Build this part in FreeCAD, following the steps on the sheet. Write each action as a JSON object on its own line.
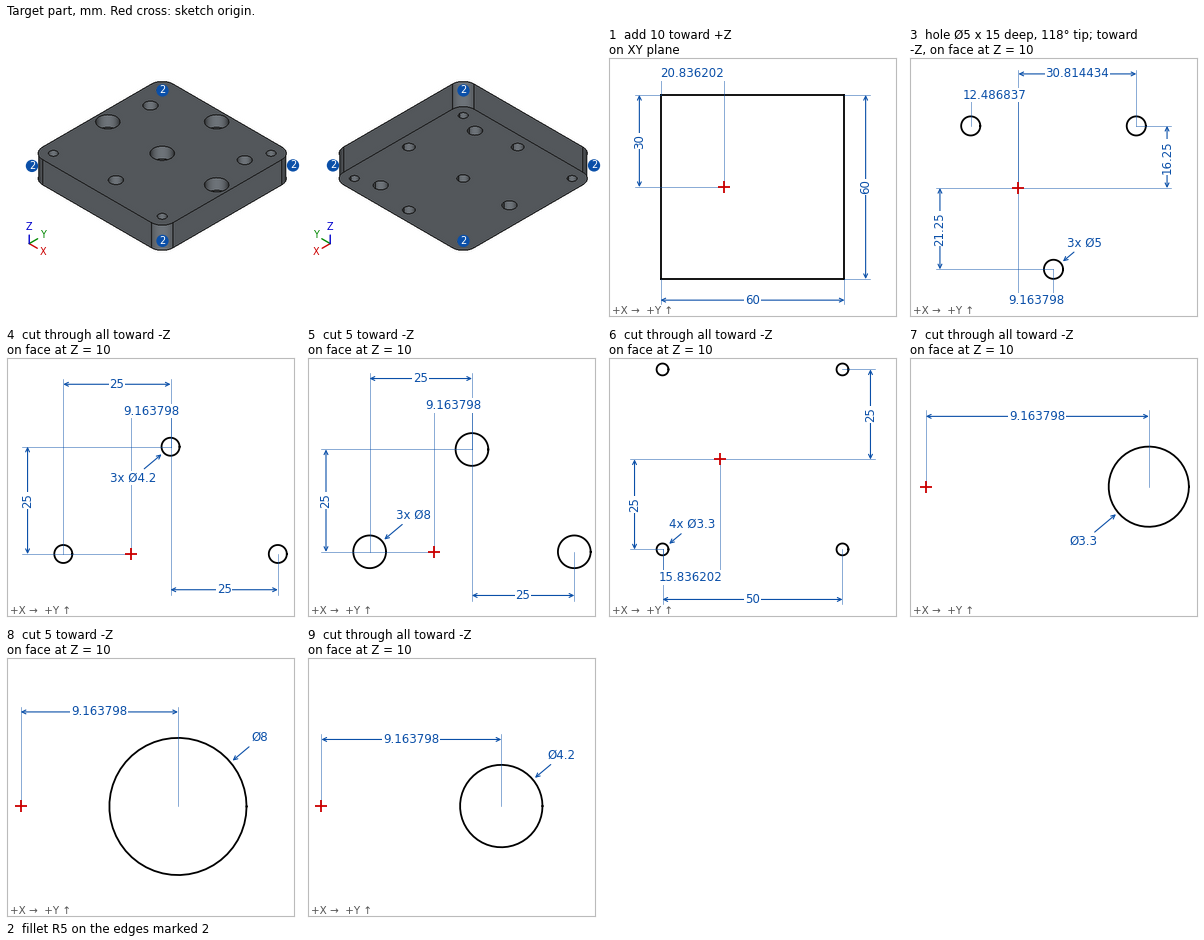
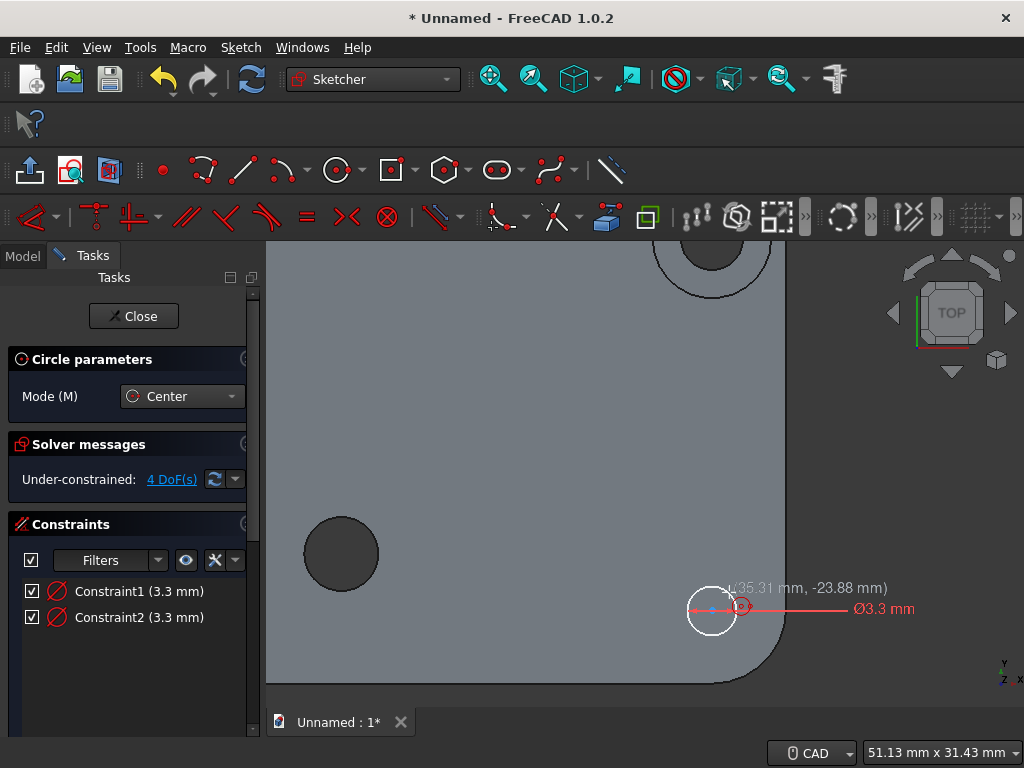
{"action": "scroll", "coordinate": [713, 611], "scroll_direction": "down", "scroll_amount": 5}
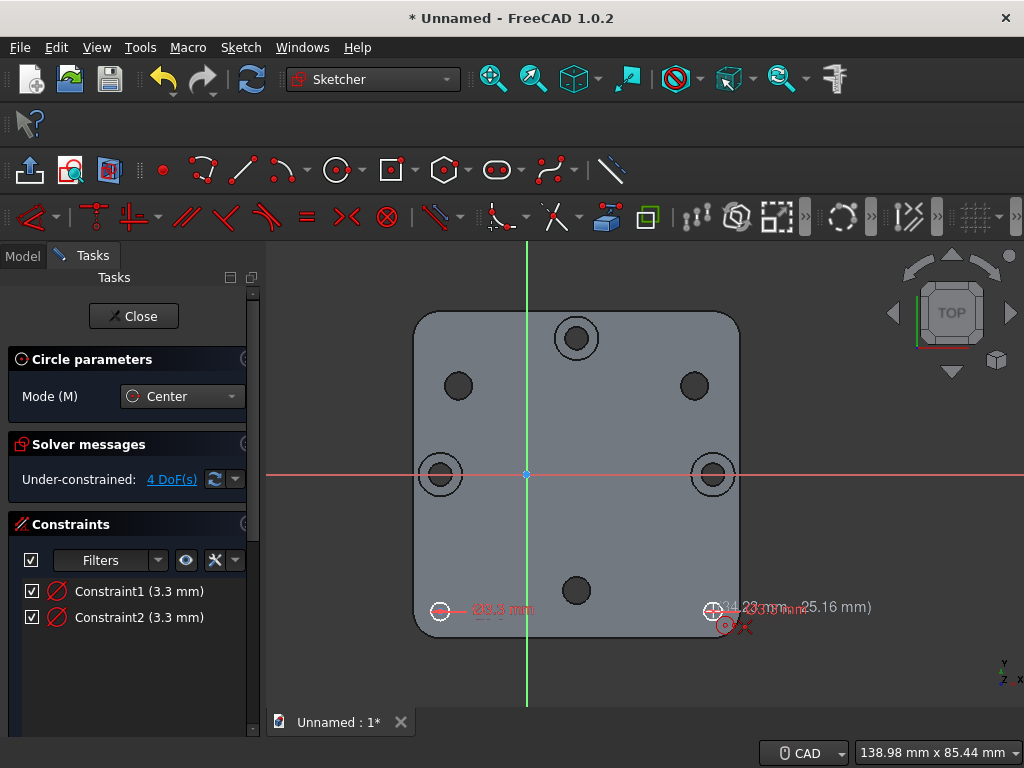
{"action": "scroll", "coordinate": [713, 338], "scroll_direction": "up", "scroll_amount": 5}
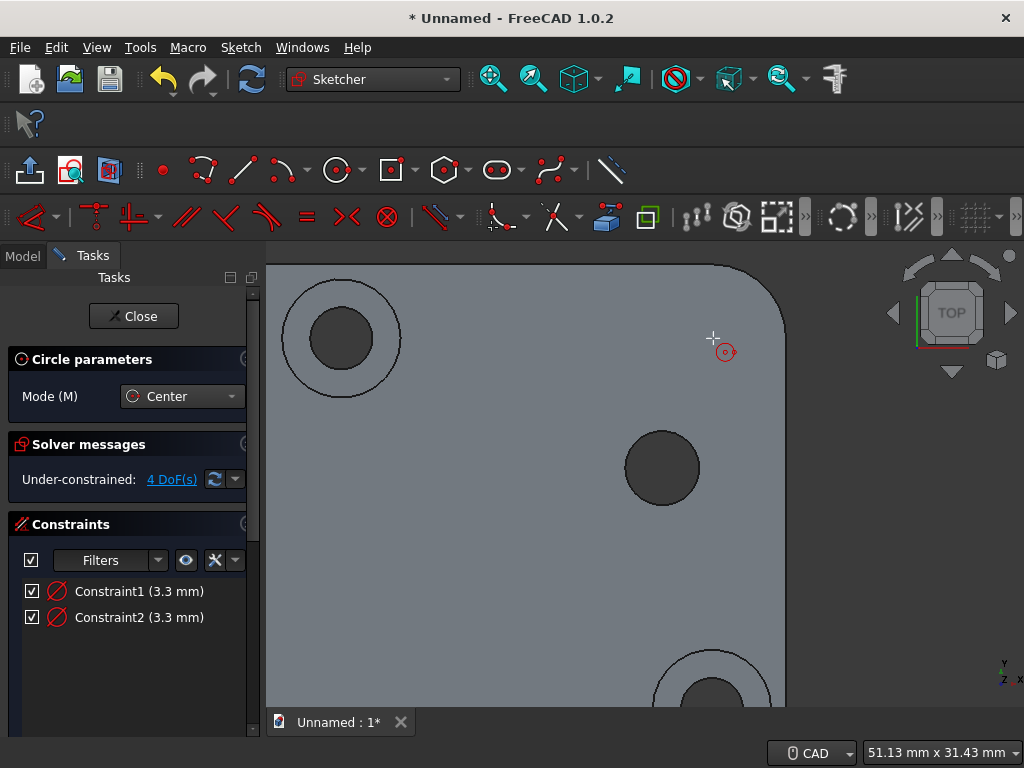
{"action": "left_click", "coordinate": [712, 338]}
{"action": "mouse_move", "coordinate": [729, 321]}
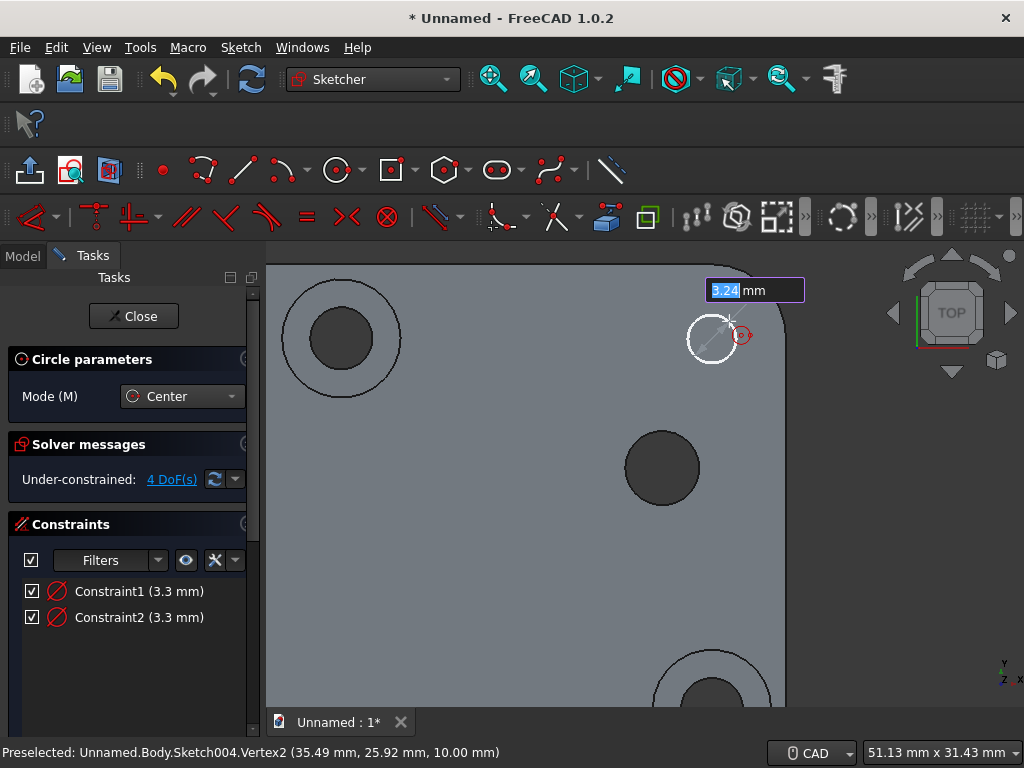
{"action": "type", "text": "3.3"}
{"action": "key", "text": "Return"}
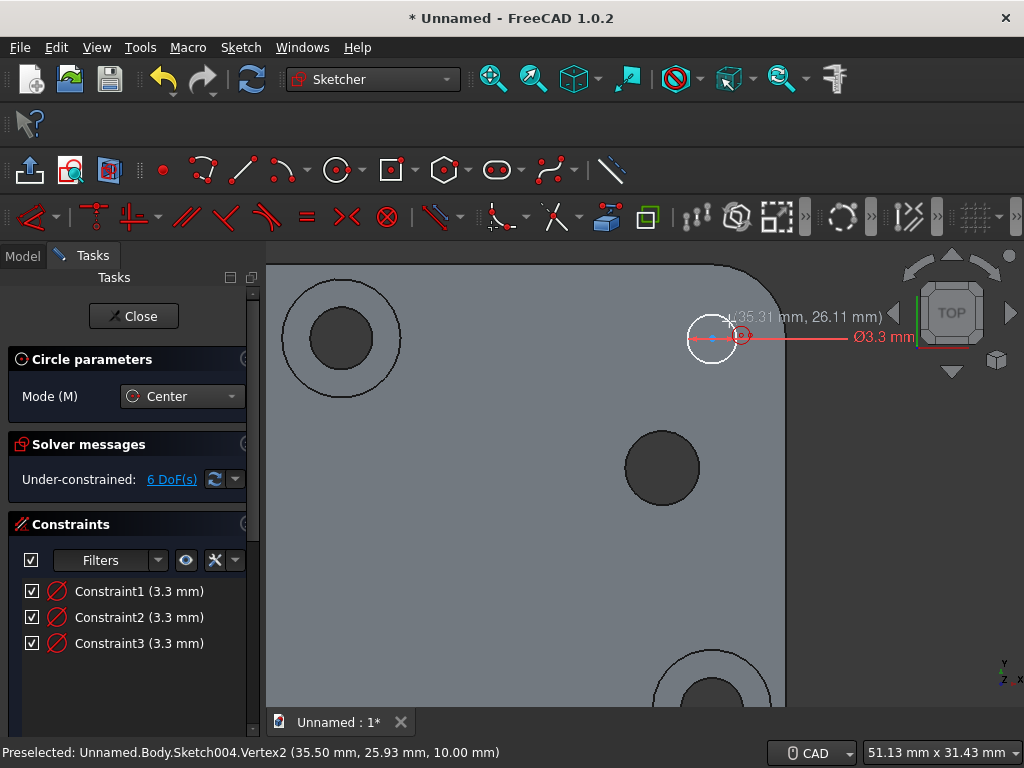
{"action": "scroll", "coordinate": [713, 337], "scroll_direction": "down", "scroll_amount": 5}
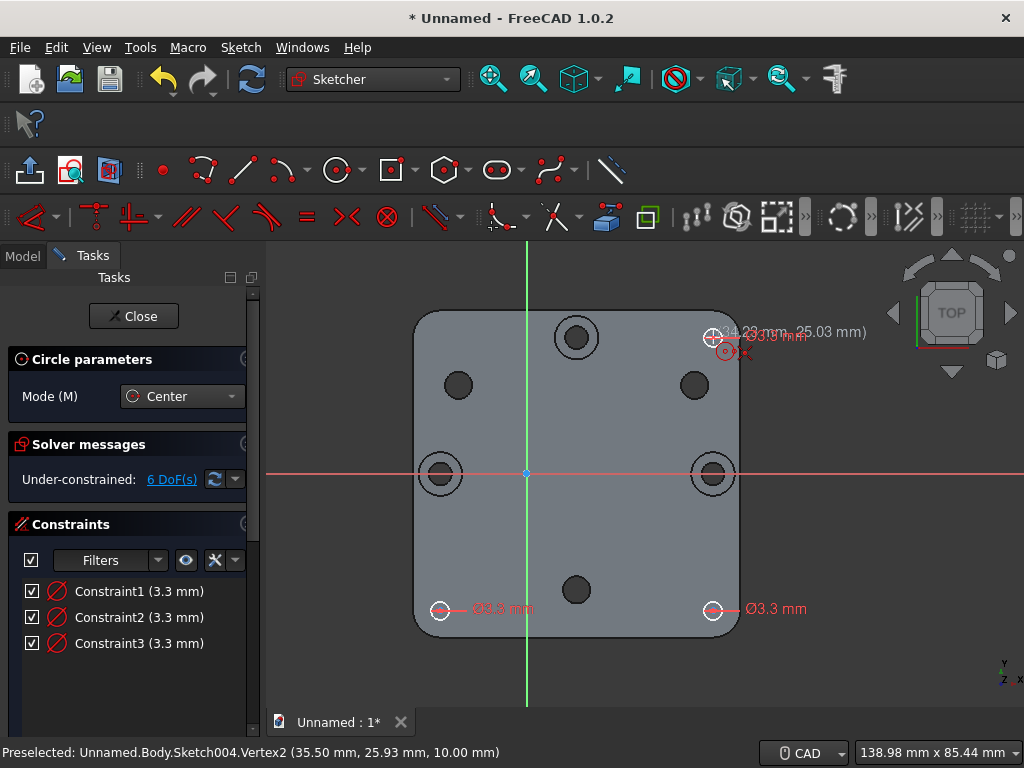
{"action": "scroll", "coordinate": [440, 338], "scroll_direction": "up", "scroll_amount": 5}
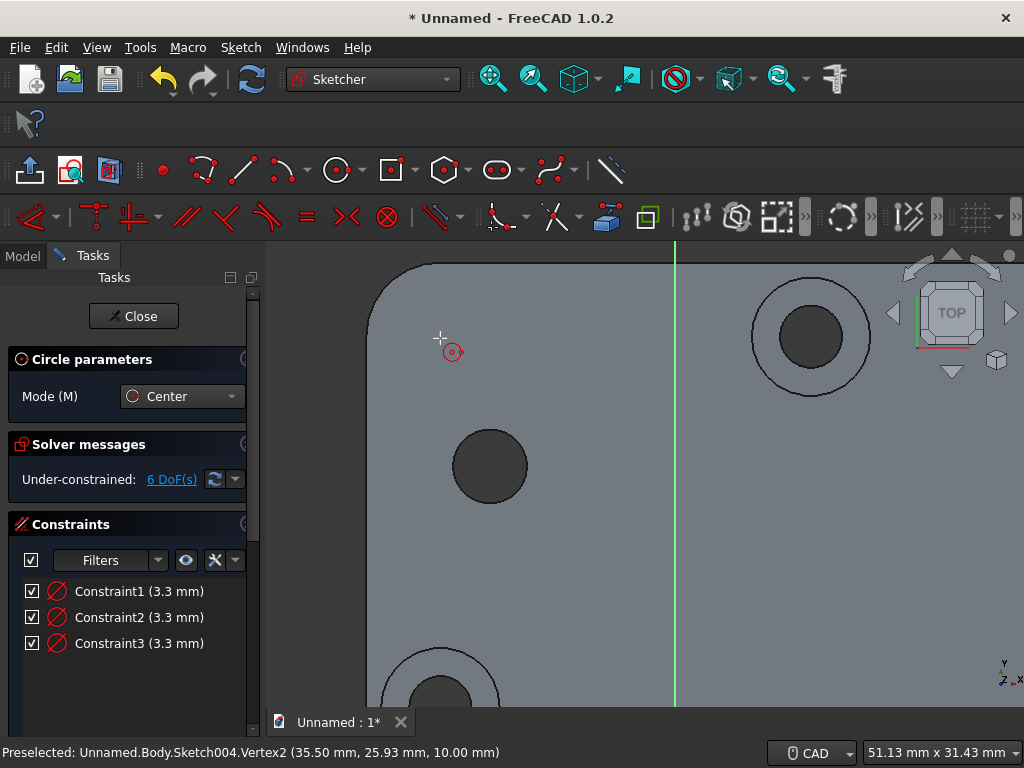
{"action": "left_click", "coordinate": [440, 337]}
{"action": "mouse_move", "coordinate": [458, 319]}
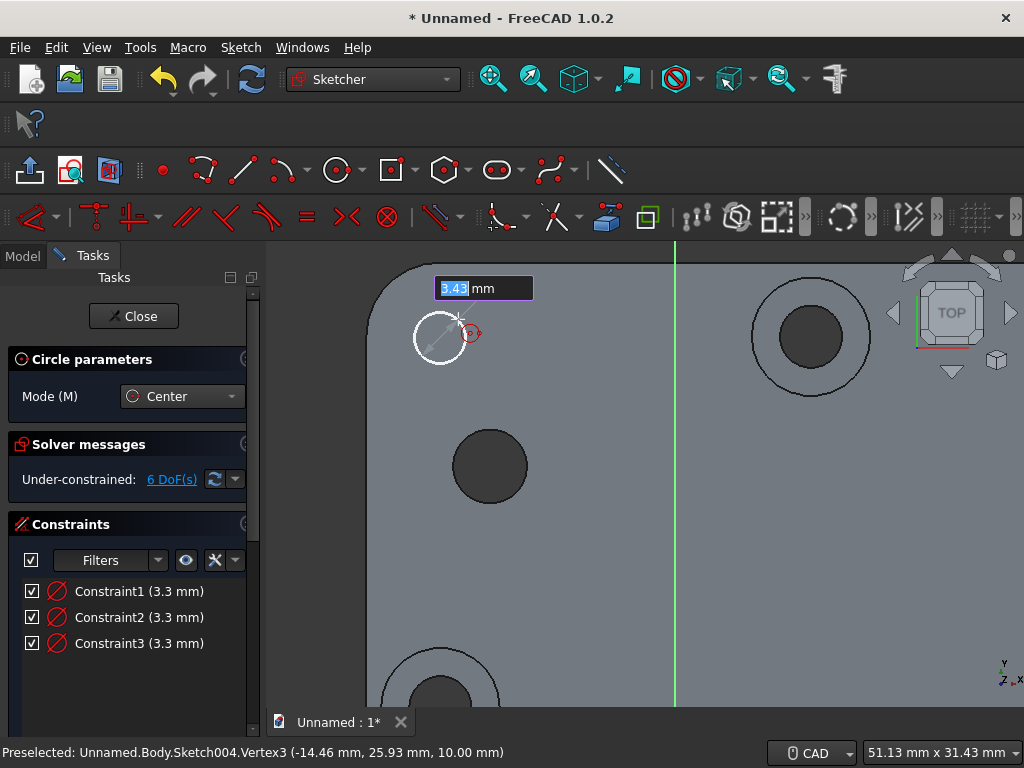
{"action": "type", "text": "3.3"}
{"action": "key", "text": "Return"}
{"action": "key", "text": "Escape"}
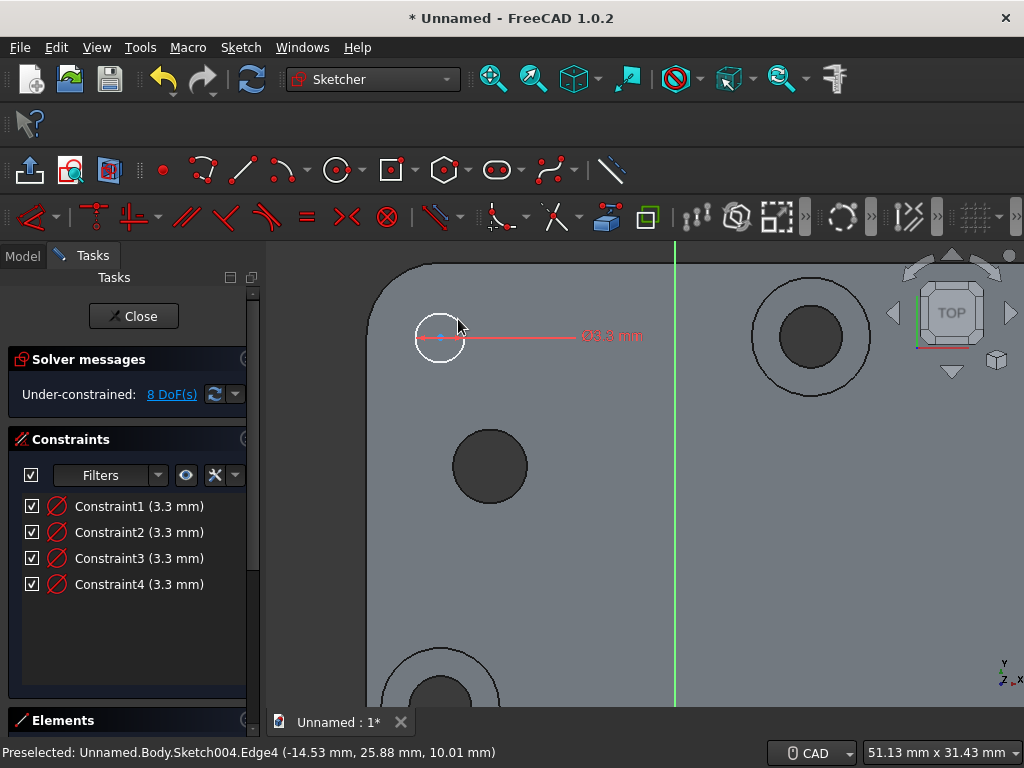
{"action": "scroll", "coordinate": [440, 338], "scroll_direction": "down", "scroll_amount": 5}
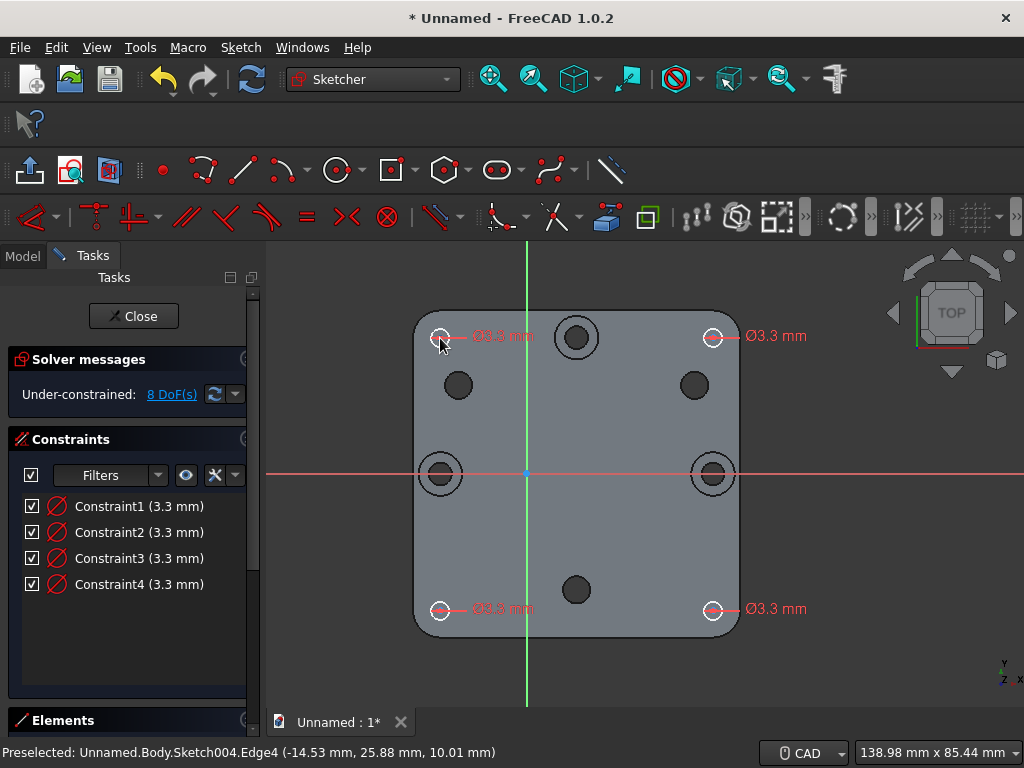
{"action": "left_click", "coordinate": [440, 611]}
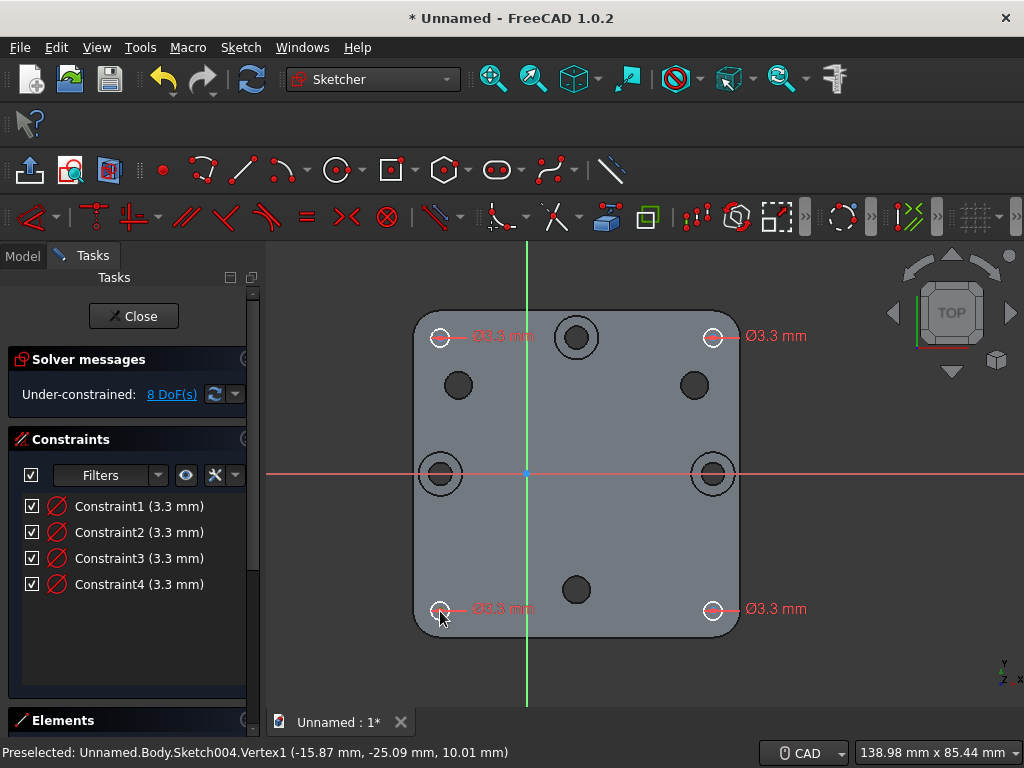
{"action": "left_click", "coordinate": [713, 611]}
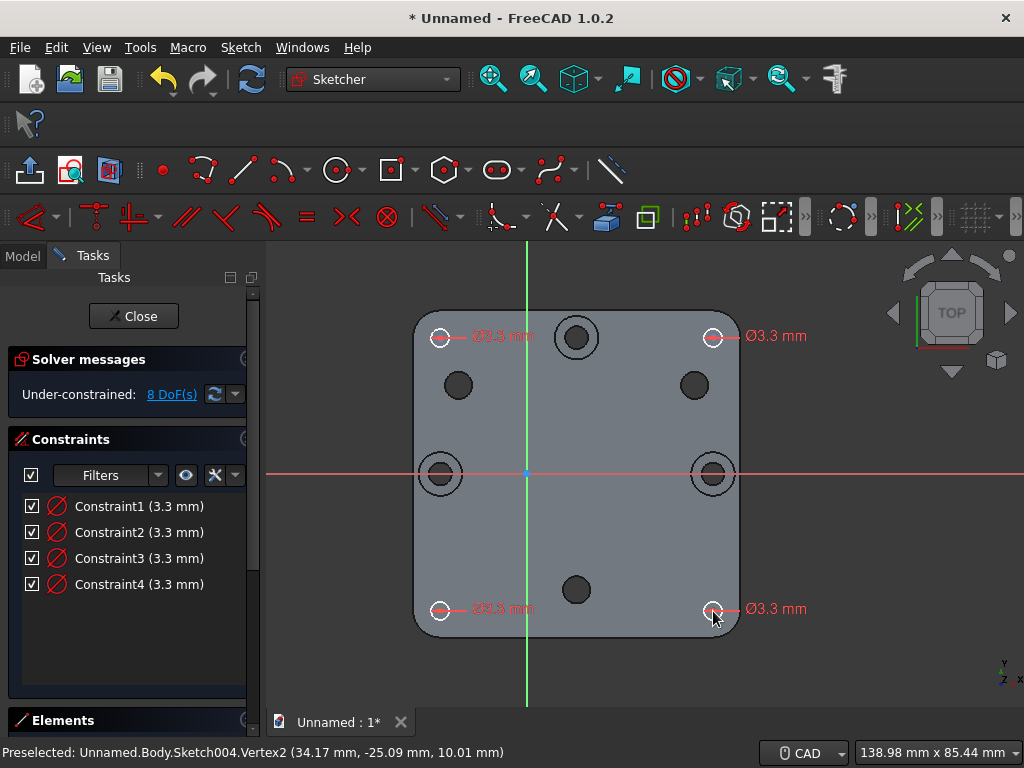
{"action": "left_click", "coordinate": [160, 218]}